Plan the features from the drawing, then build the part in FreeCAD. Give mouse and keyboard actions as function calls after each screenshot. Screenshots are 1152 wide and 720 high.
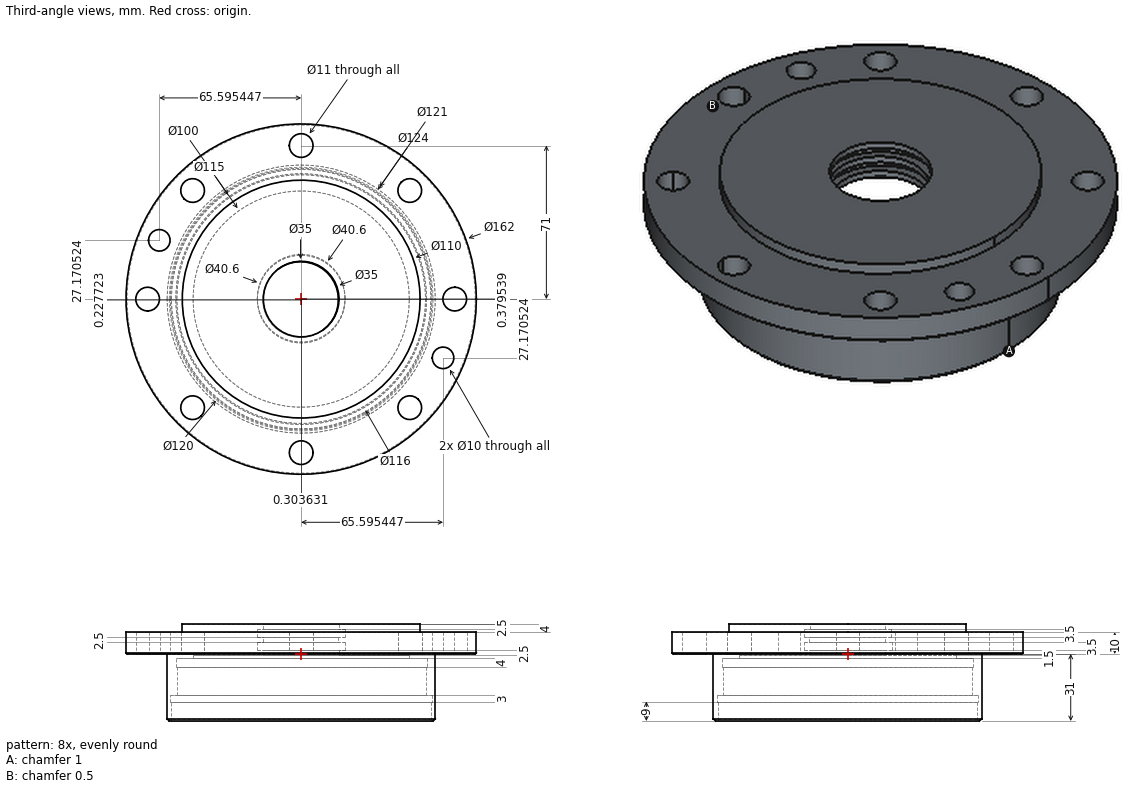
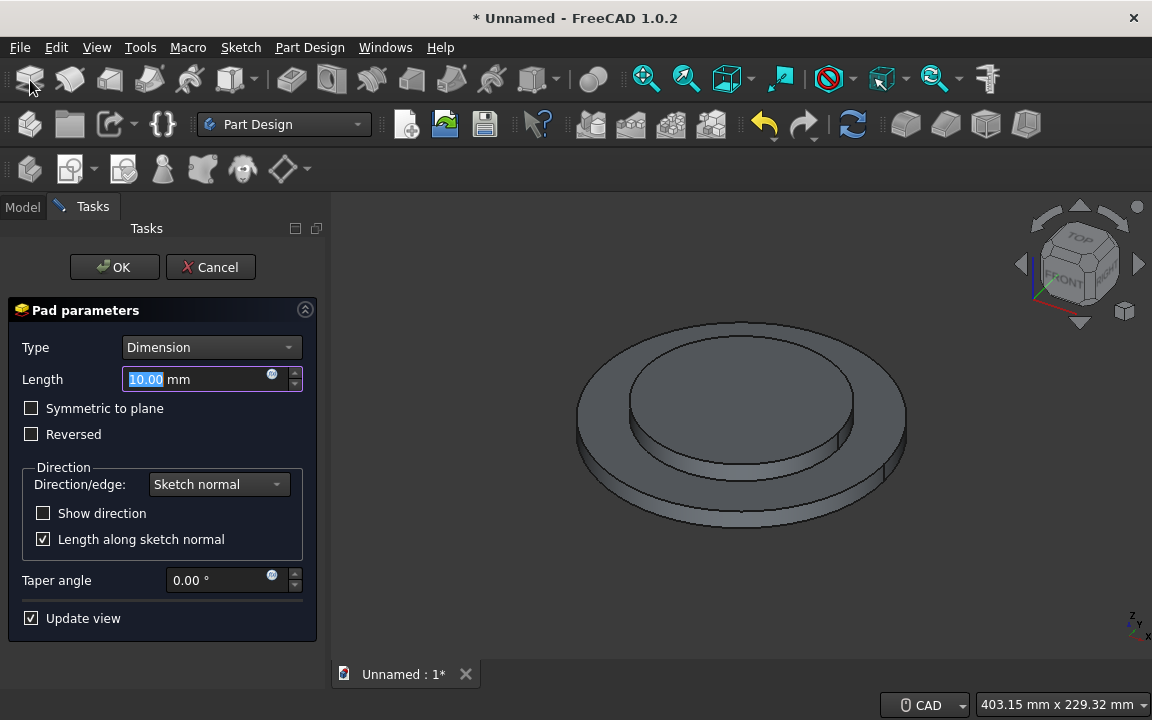
text(4)
key(Tab)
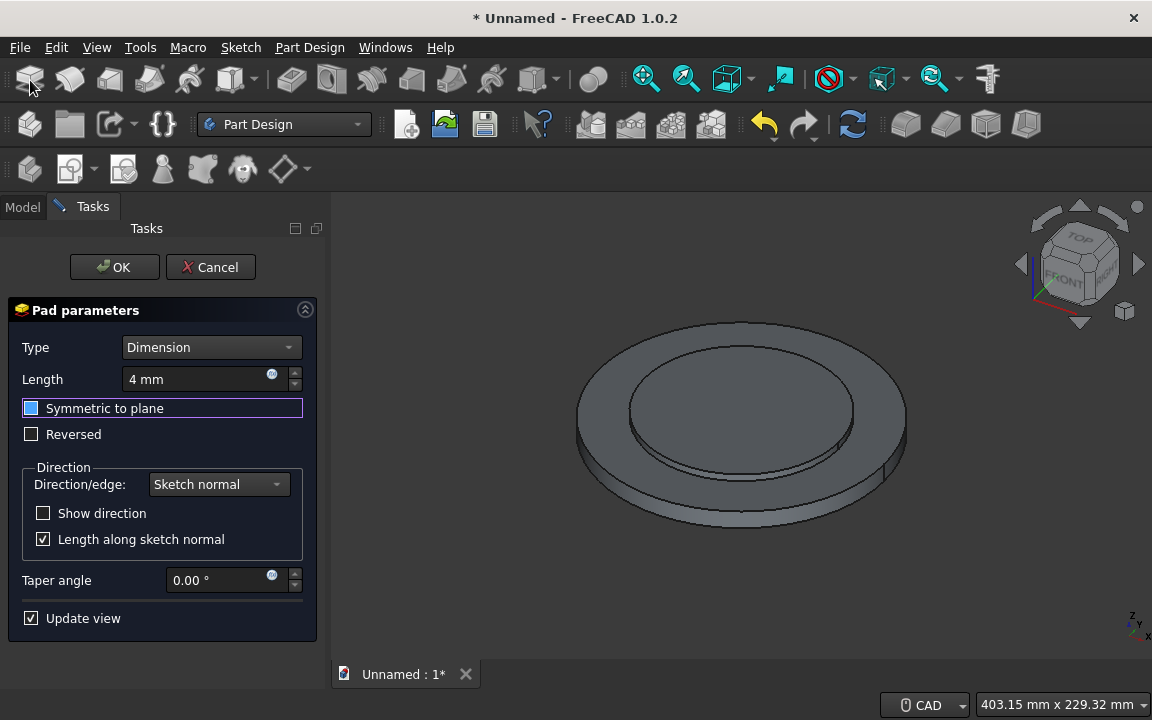
click(115, 267)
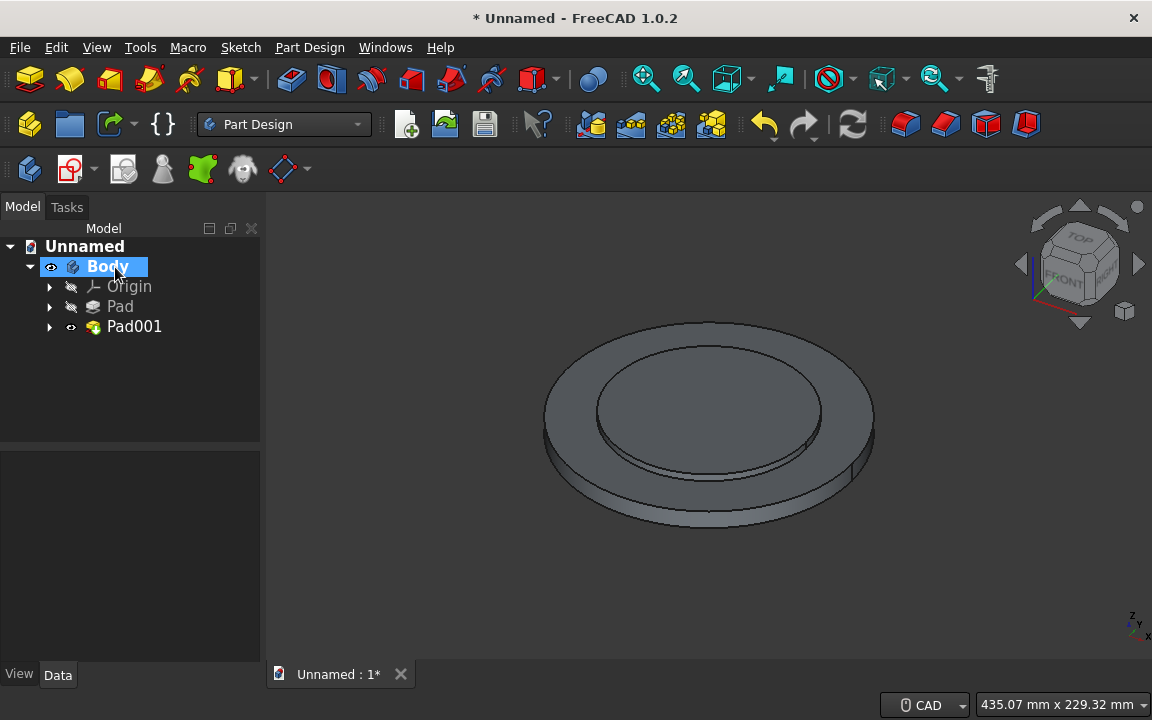
click(70, 170)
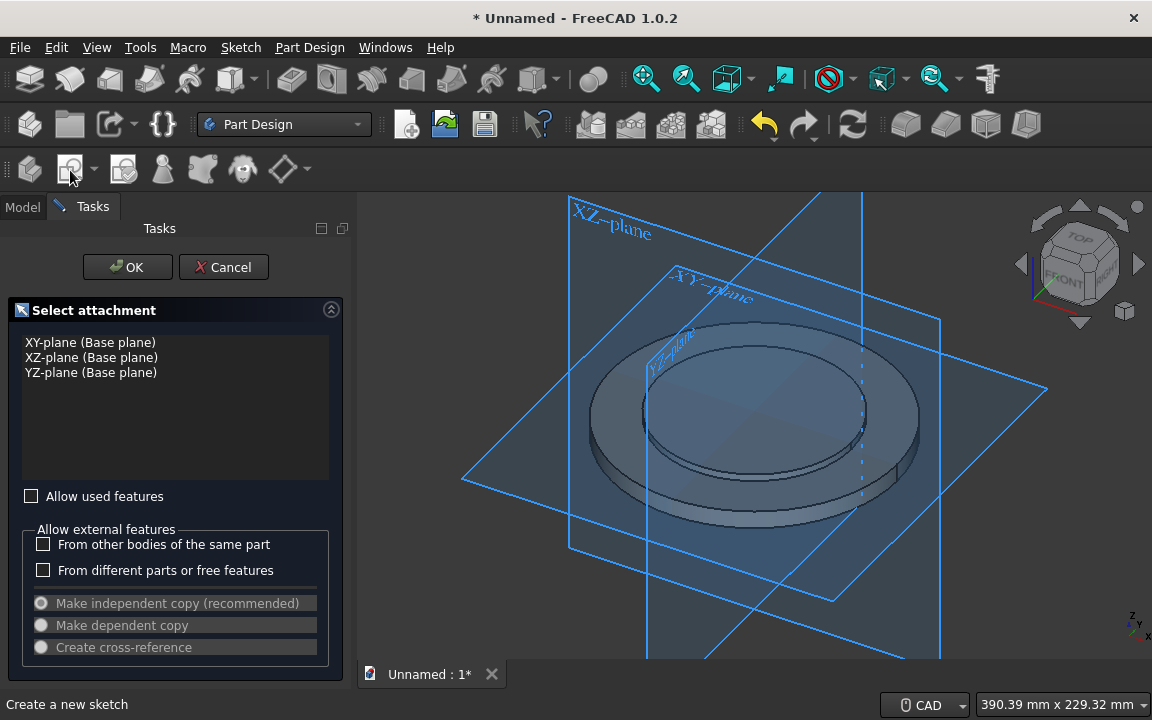
click(82, 342)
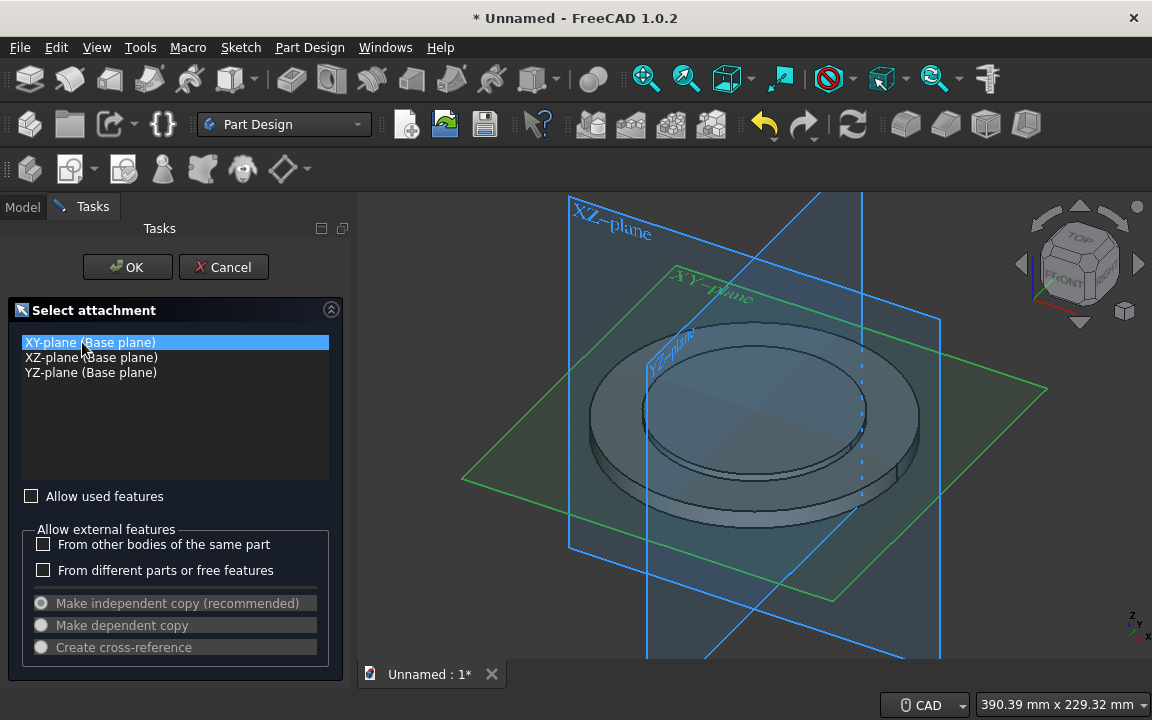
click(128, 267)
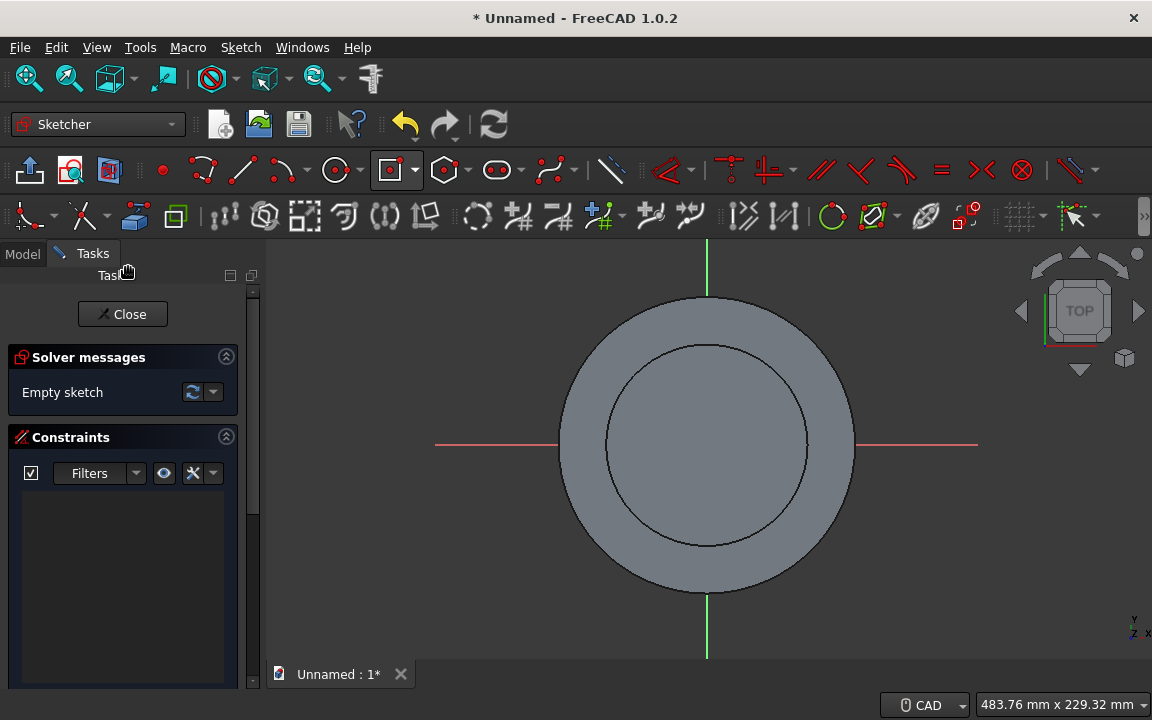
click(110, 170)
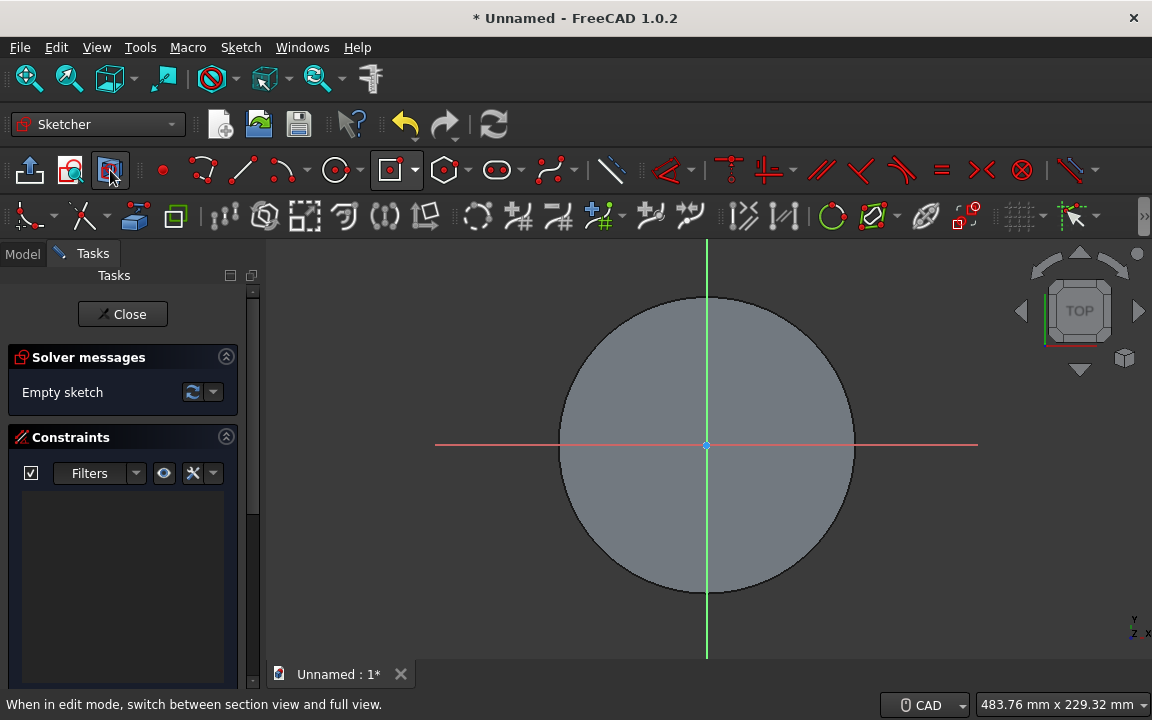
key(g)
key(c)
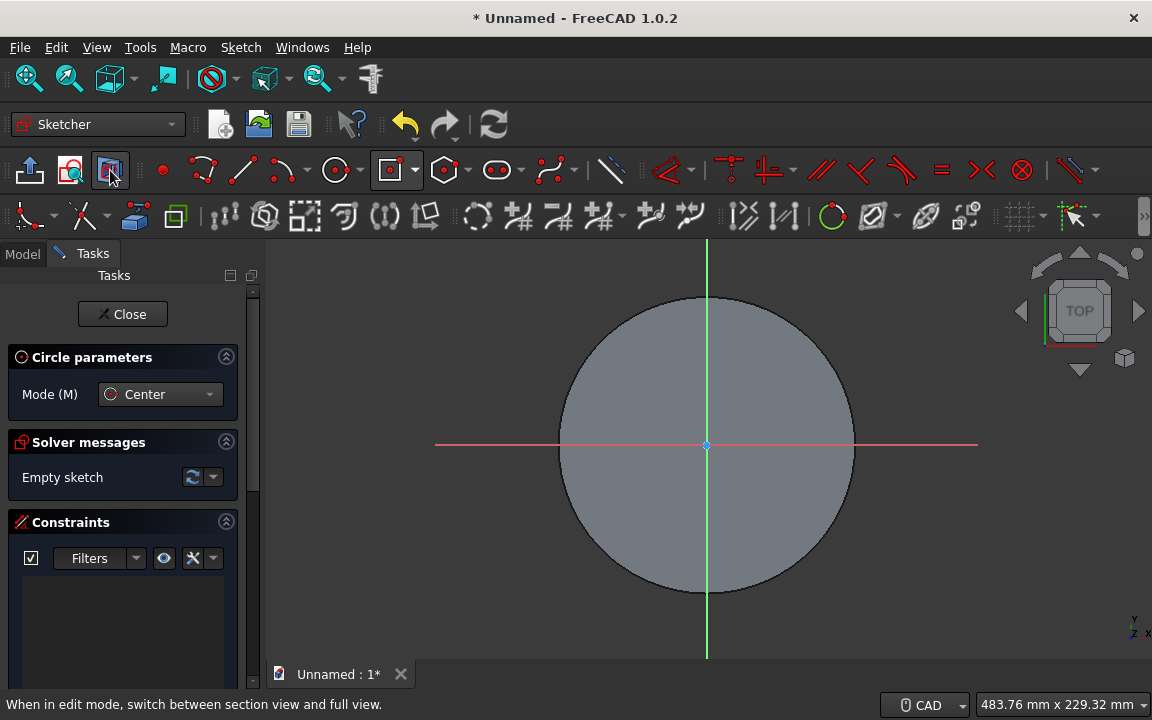
click(707, 445)
click(787, 365)
key(Escape)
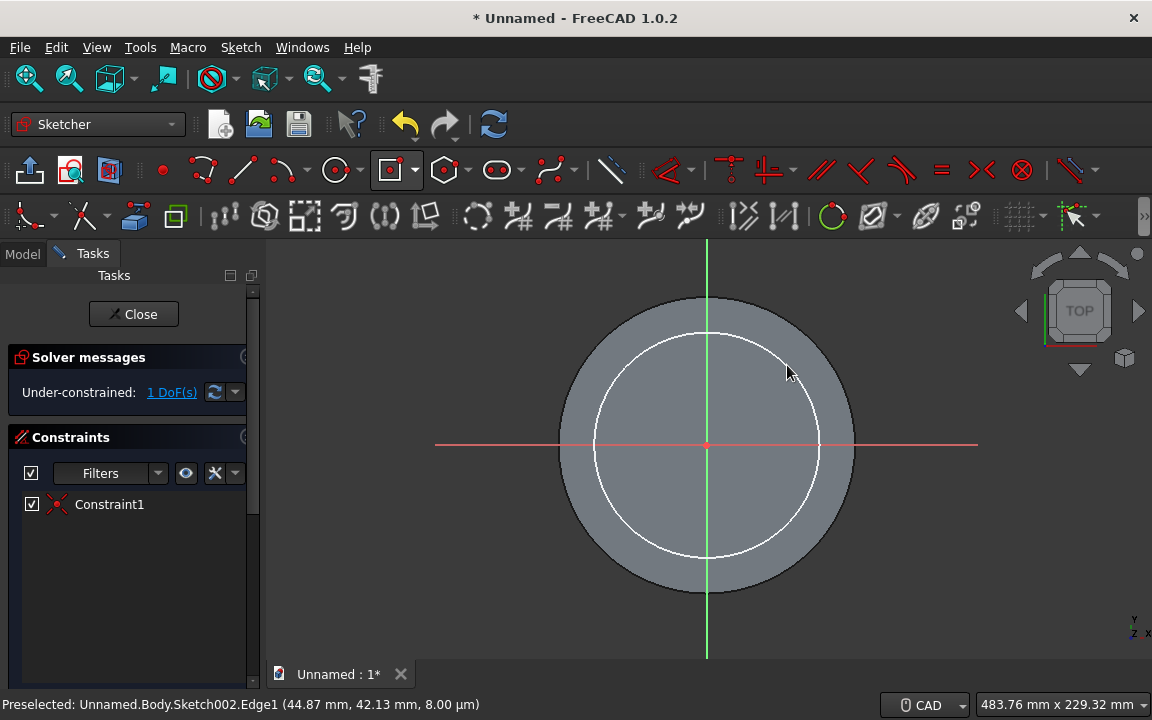
click(666, 170)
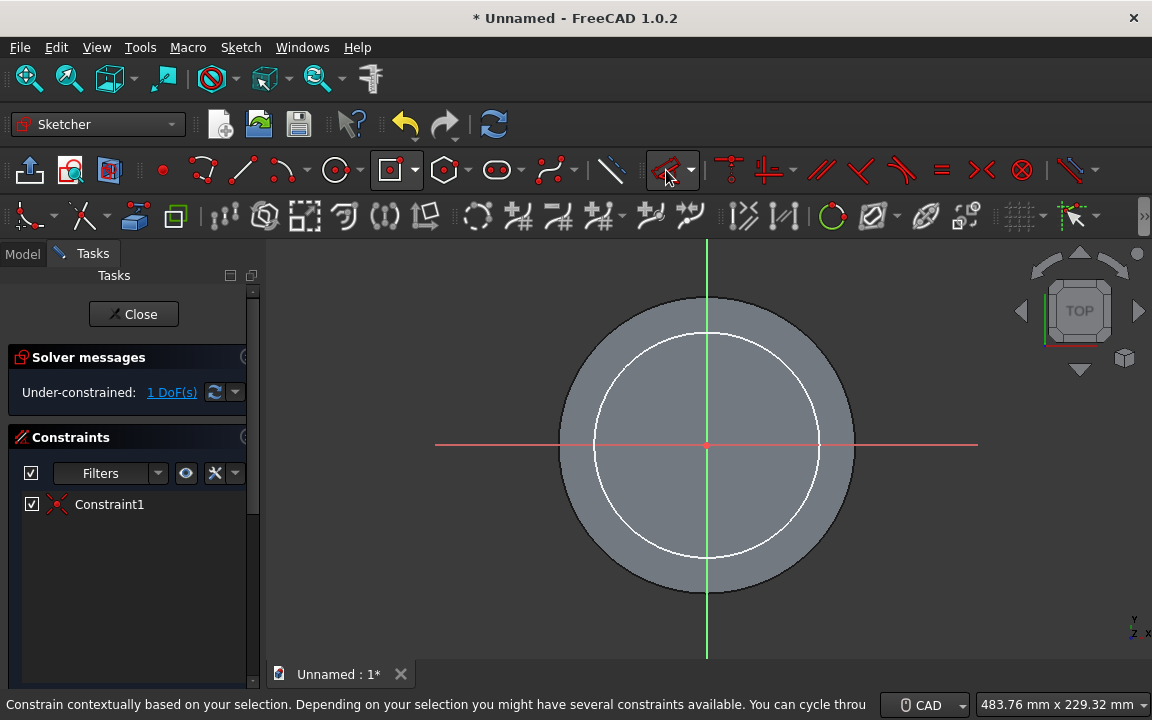
click(786, 365)
click(808, 342)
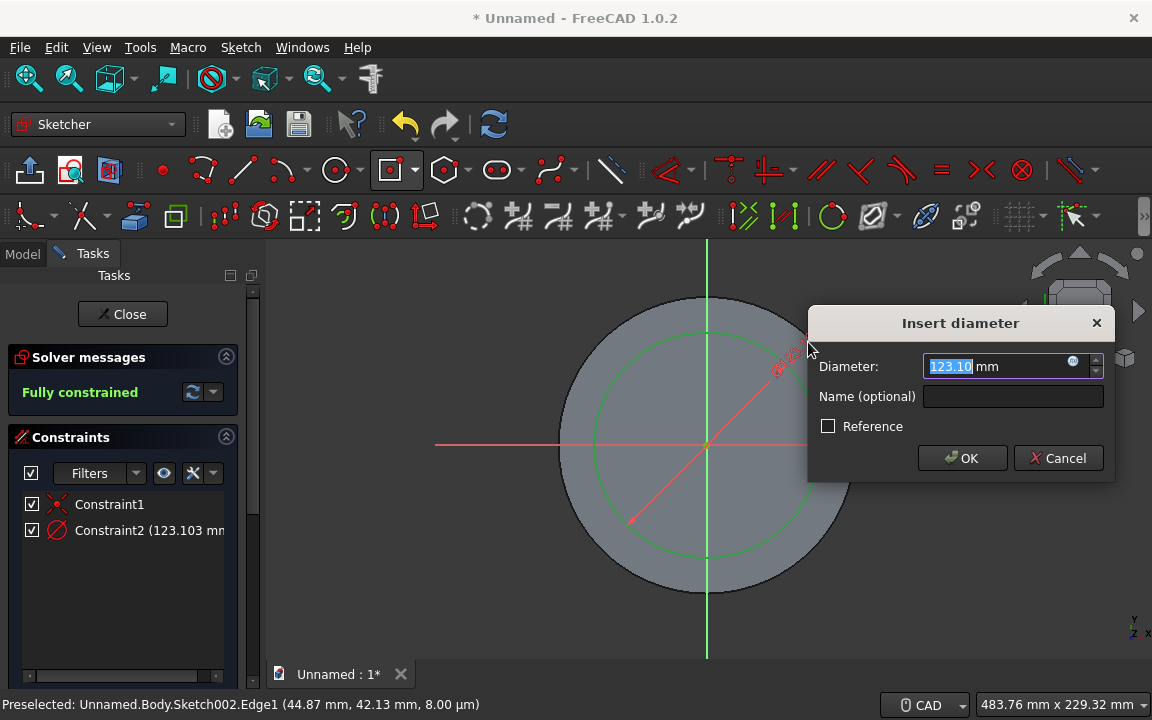
text(124)
key(Return)
key(Escape)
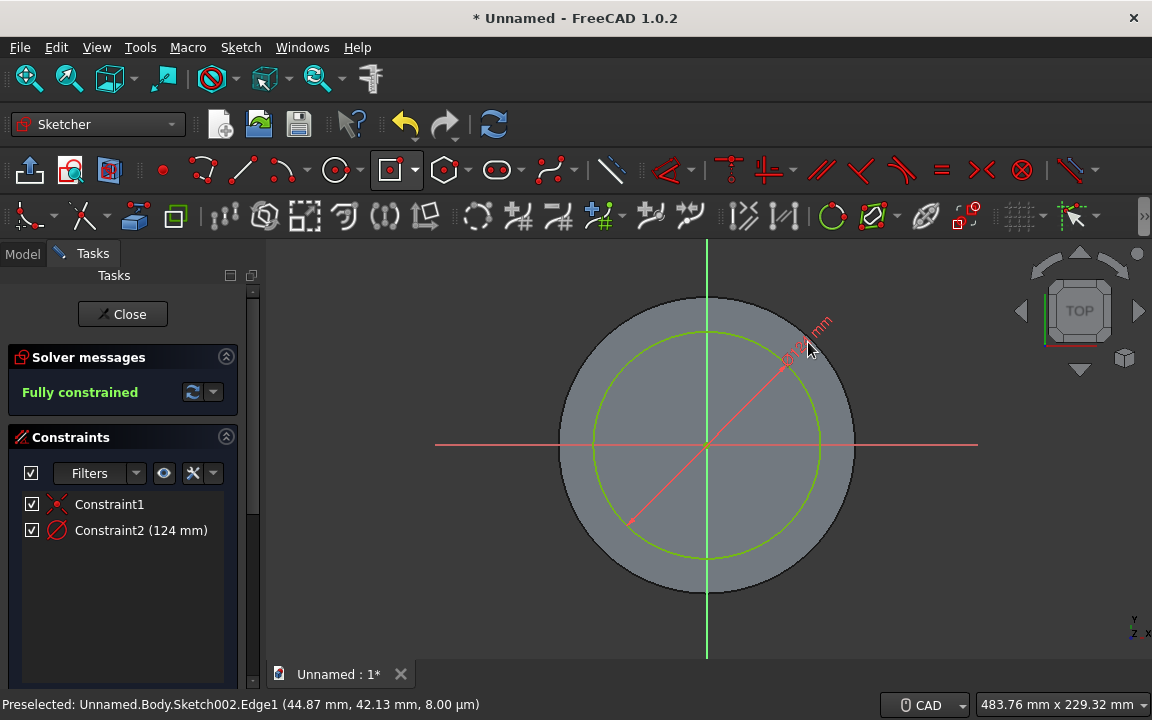
click(123, 314)